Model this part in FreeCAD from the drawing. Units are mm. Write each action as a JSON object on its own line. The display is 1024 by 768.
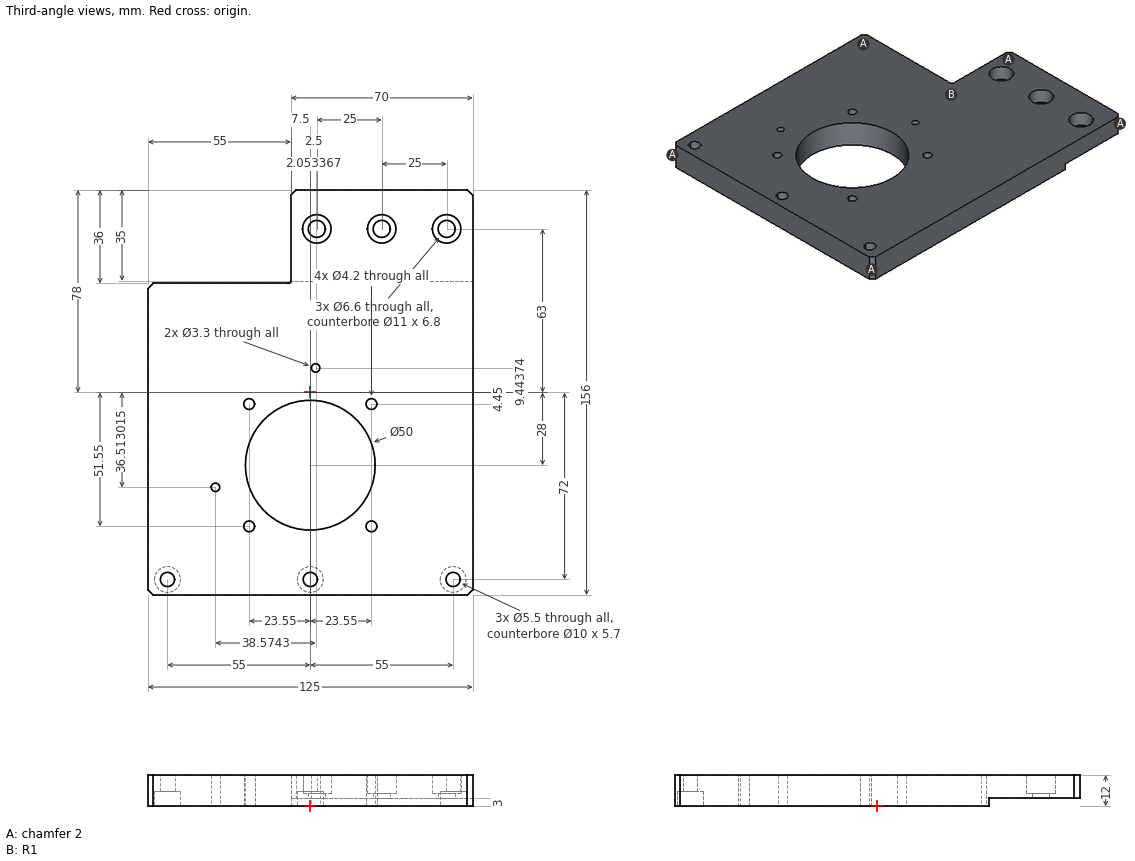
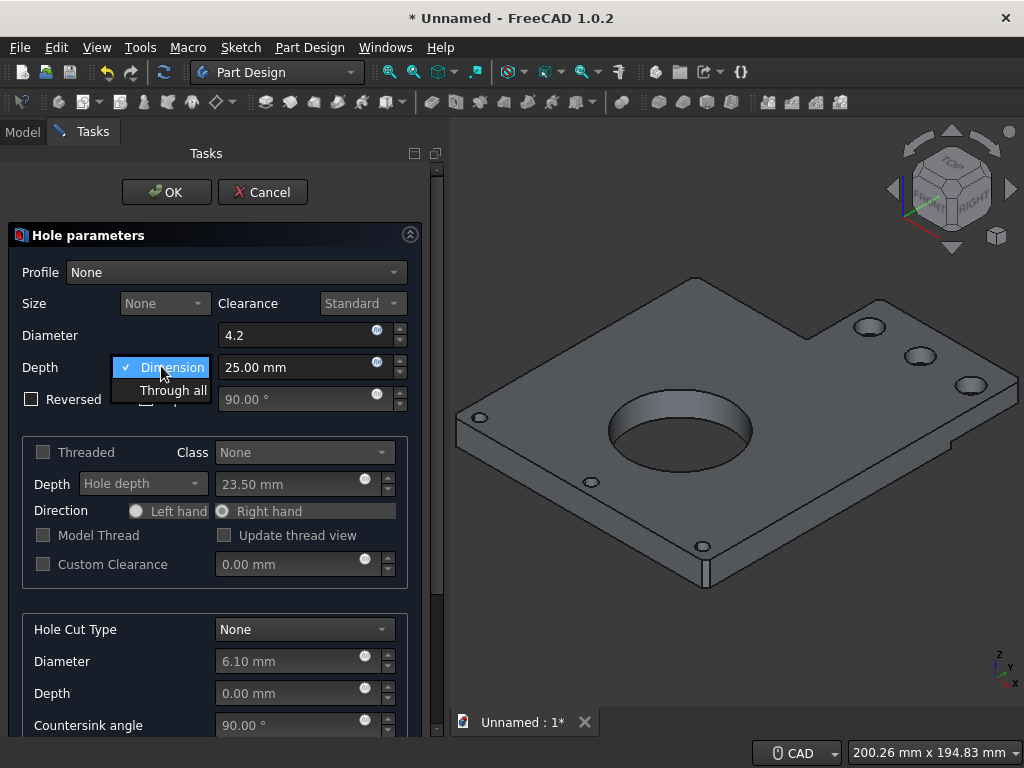
{"action": "left_click", "coordinate": [160, 390]}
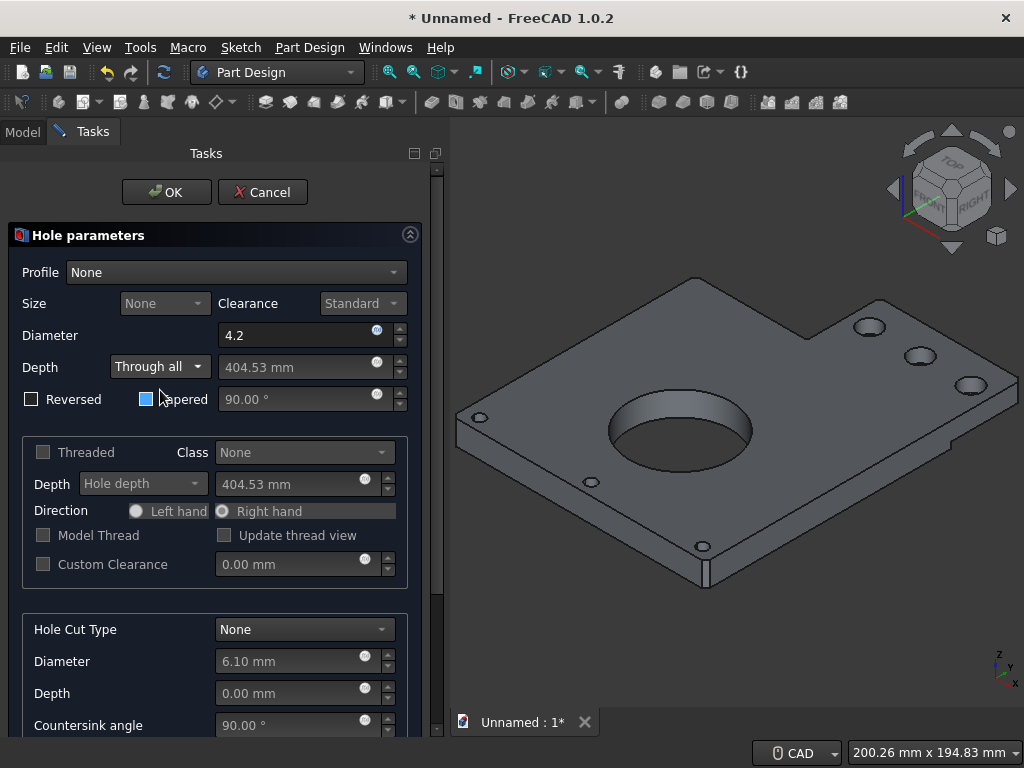
{"action": "left_click", "coordinate": [30, 399]}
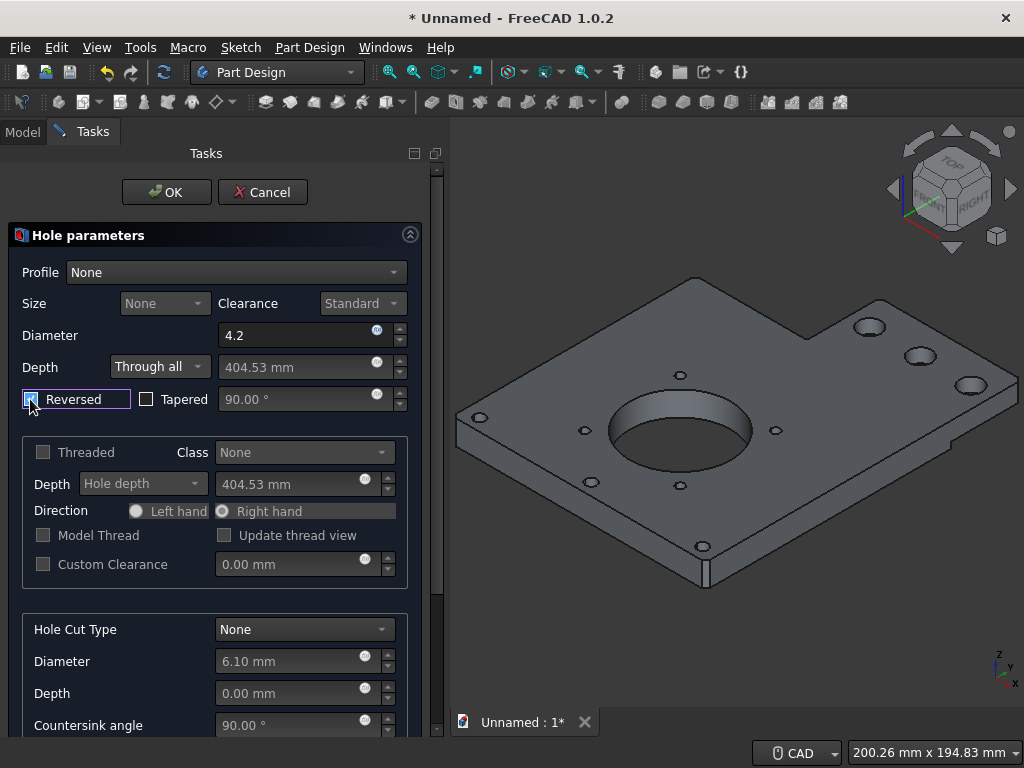
{"action": "left_click", "coordinate": [167, 192]}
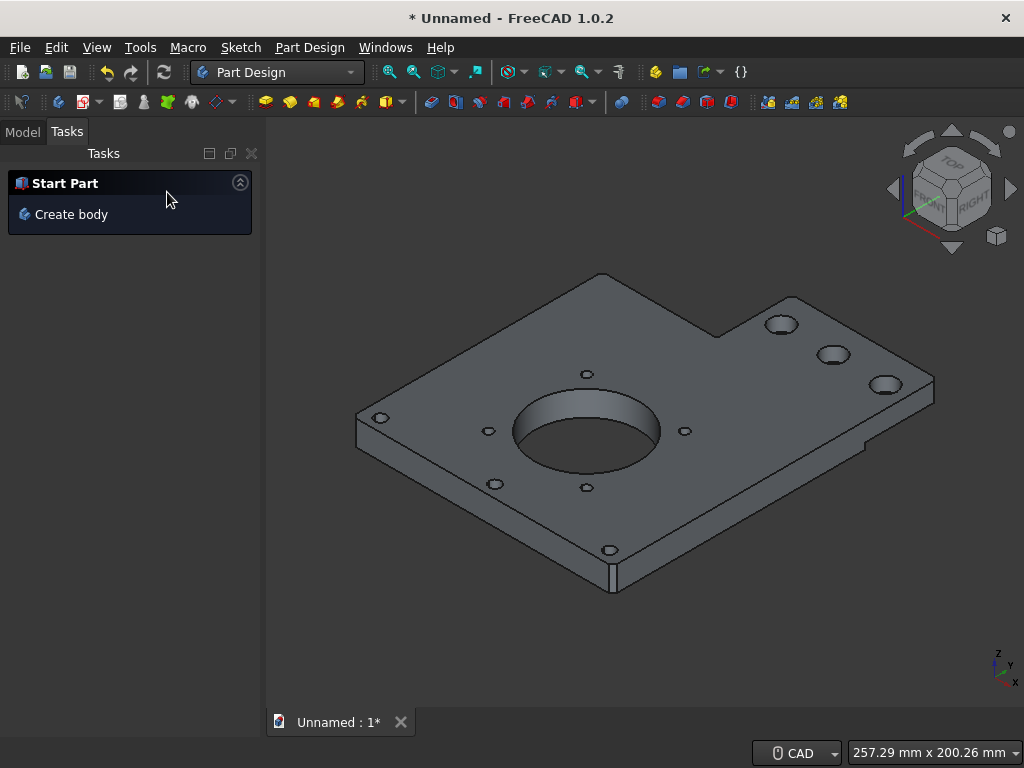
{"action": "left_click", "coordinate": [766, 413]}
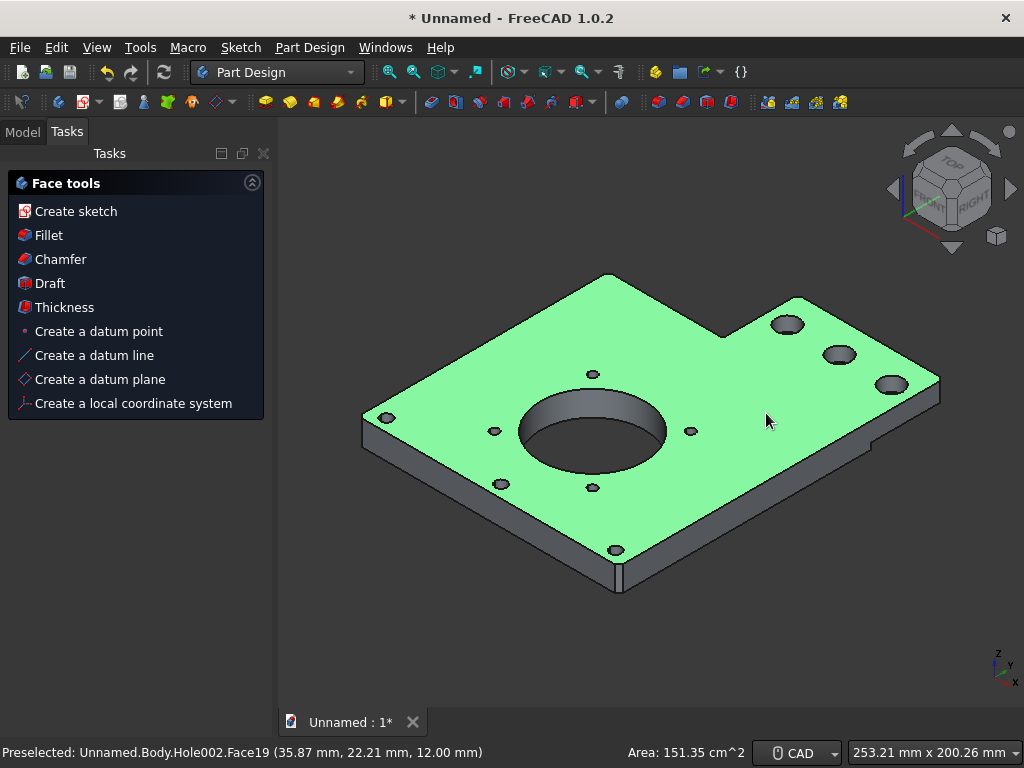
{"action": "left_click", "coordinate": [84, 102]}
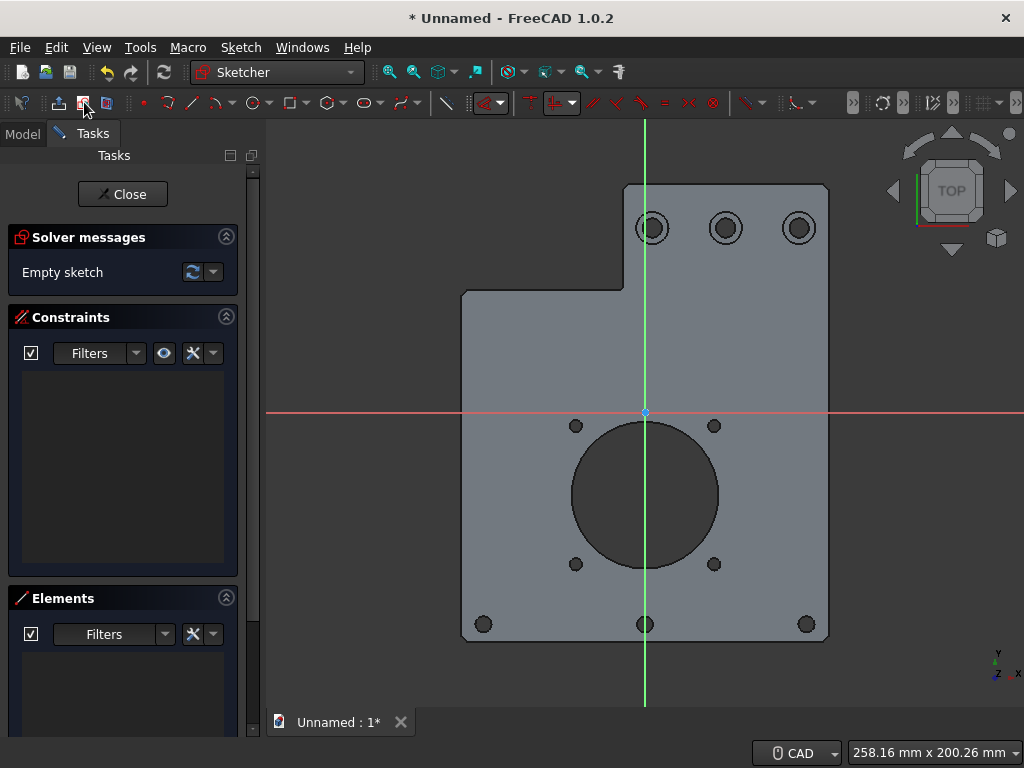
{"action": "scroll", "coordinate": [605, 476], "scroll_direction": "up", "scroll_amount": 5}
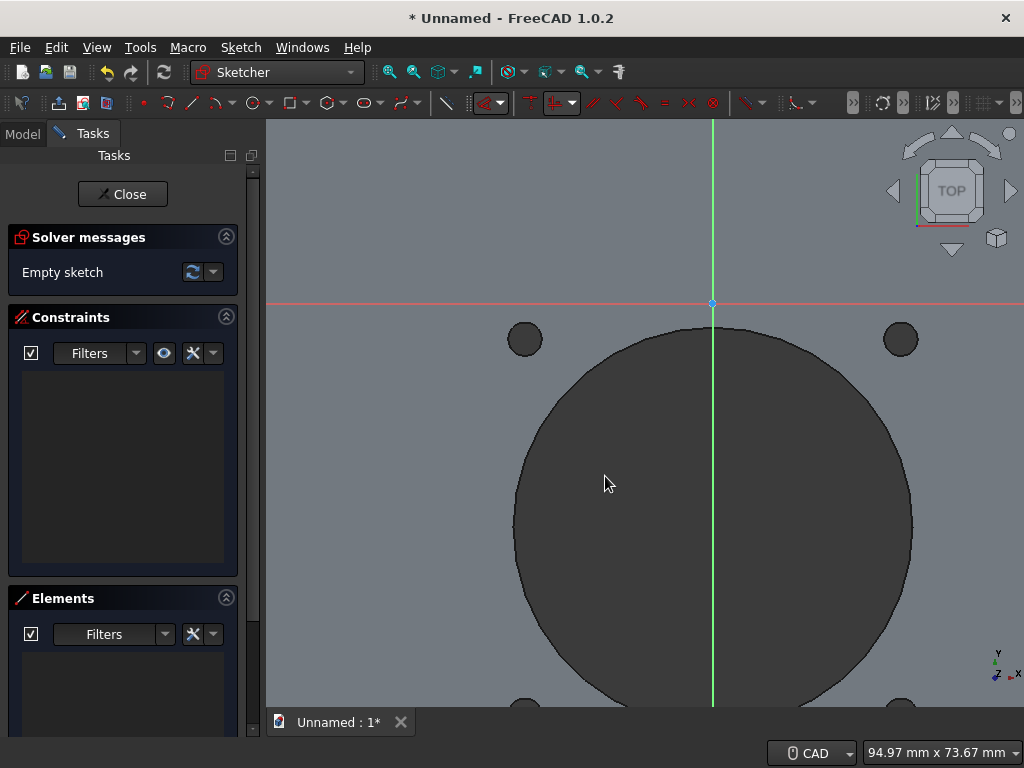
{"action": "left_click", "coordinate": [254, 104]}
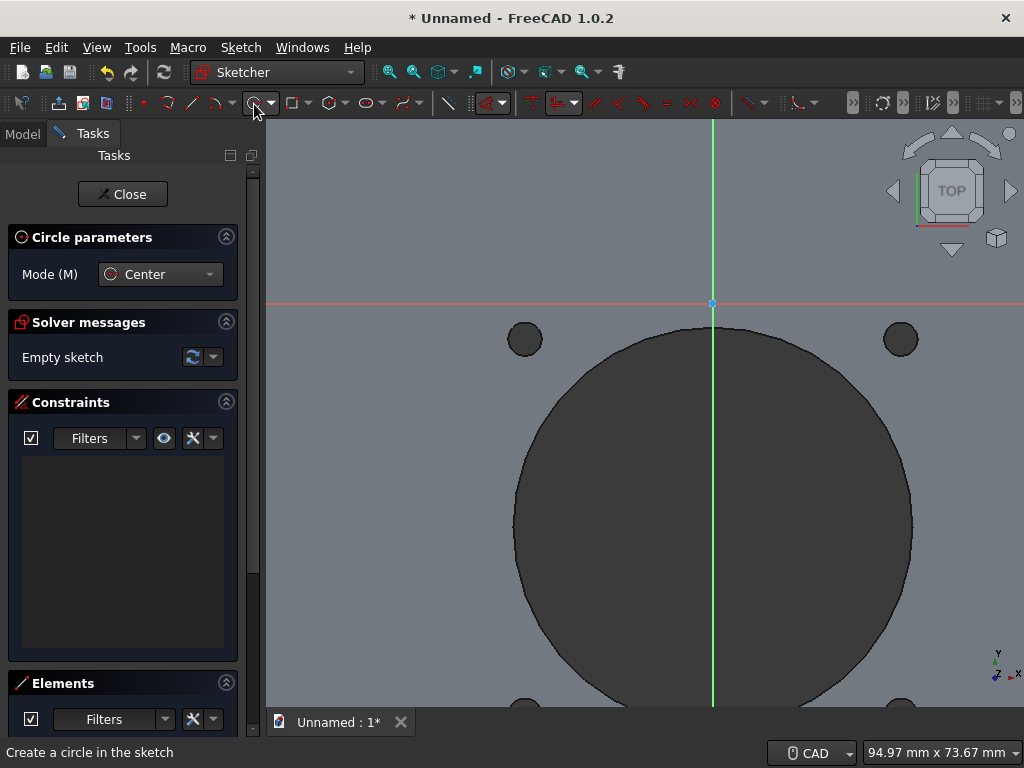
{"action": "scroll", "coordinate": [729, 228], "scroll_direction": "up", "scroll_amount": 3}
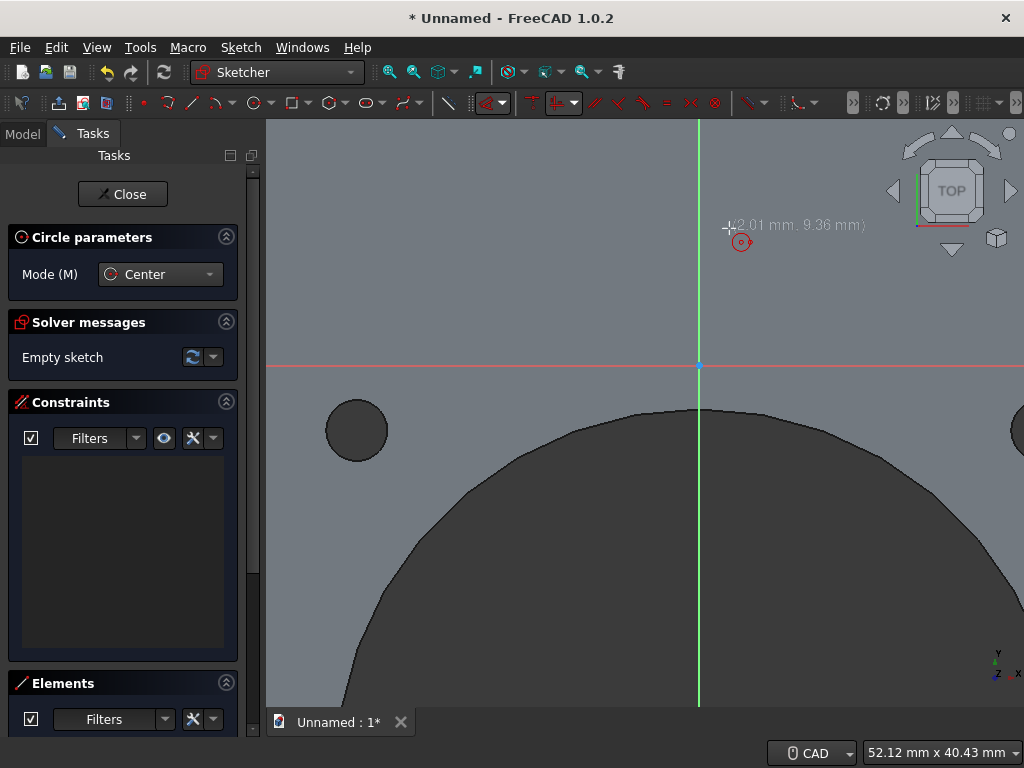
{"action": "left_click", "coordinate": [729, 228]}
{"action": "left_click", "coordinate": [746, 211]}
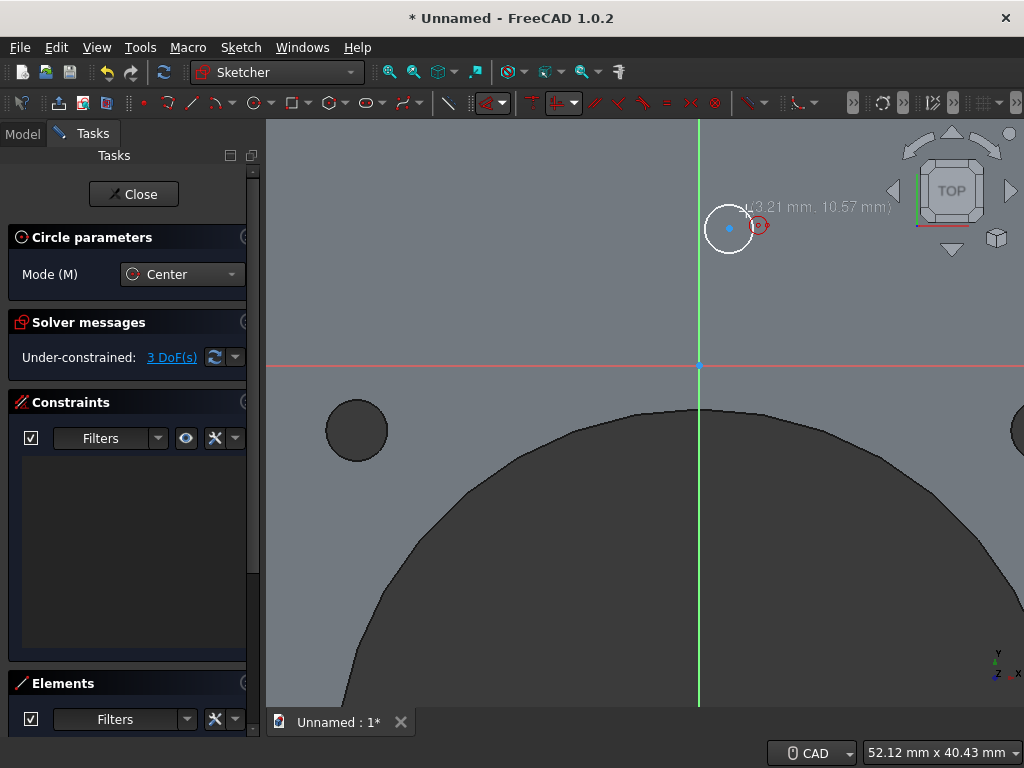
{"action": "scroll", "coordinate": [732, 231], "scroll_direction": "down", "scroll_amount": 3}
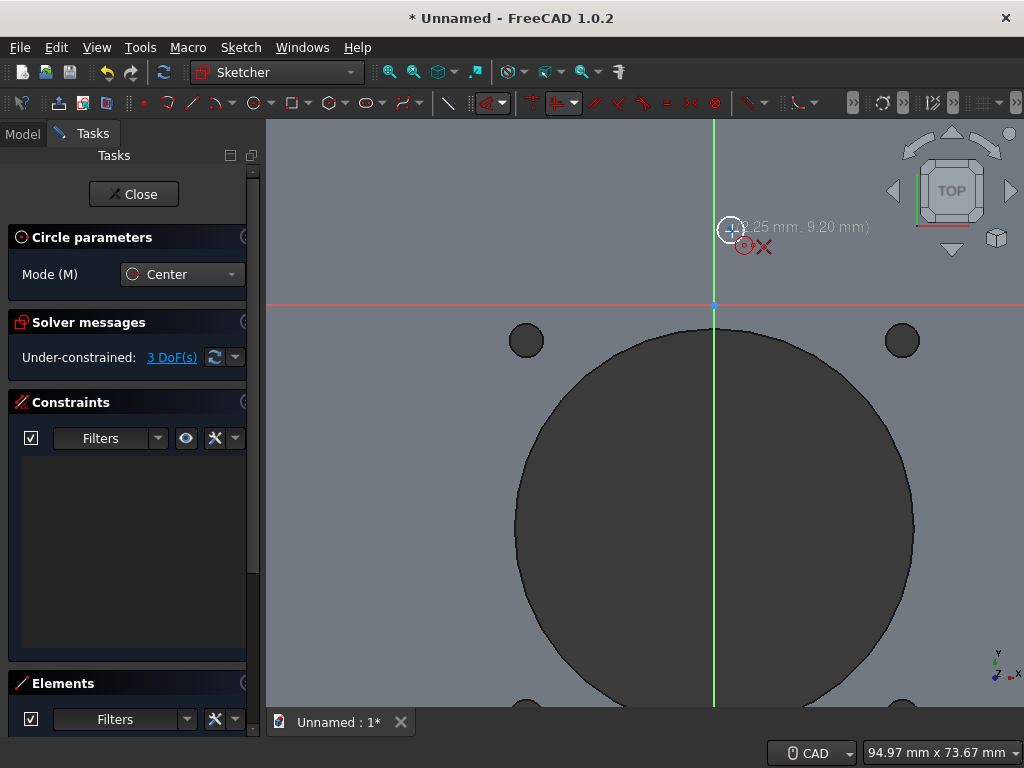
{"action": "scroll", "coordinate": [423, 596], "scroll_direction": "up", "scroll_amount": 3}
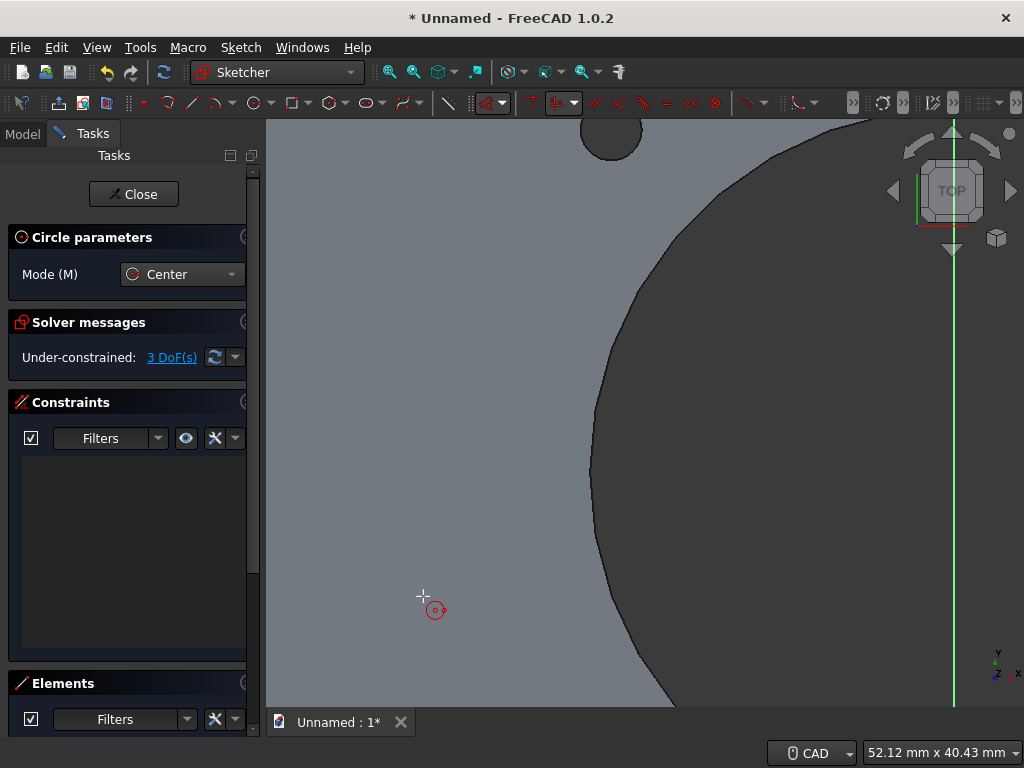
{"action": "left_click", "coordinate": [423, 596]}
{"action": "left_click", "coordinate": [439, 579]}
{"action": "key", "text": "Escape"}